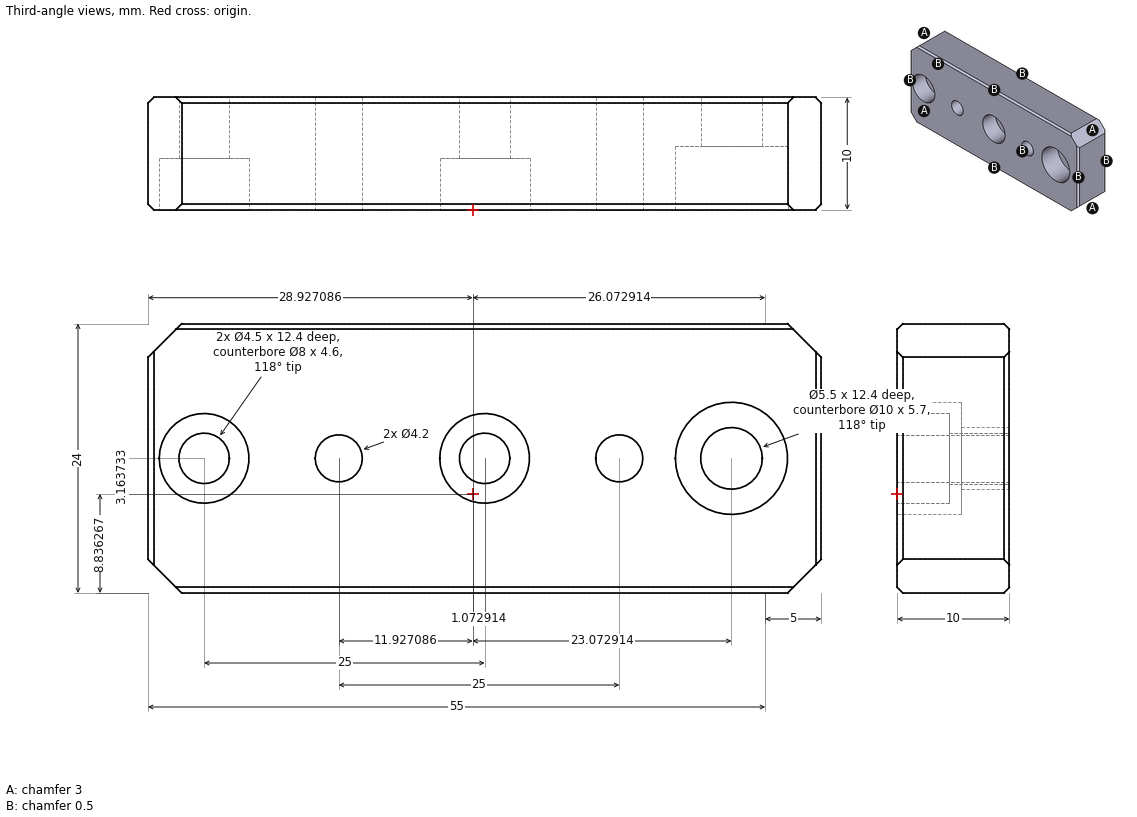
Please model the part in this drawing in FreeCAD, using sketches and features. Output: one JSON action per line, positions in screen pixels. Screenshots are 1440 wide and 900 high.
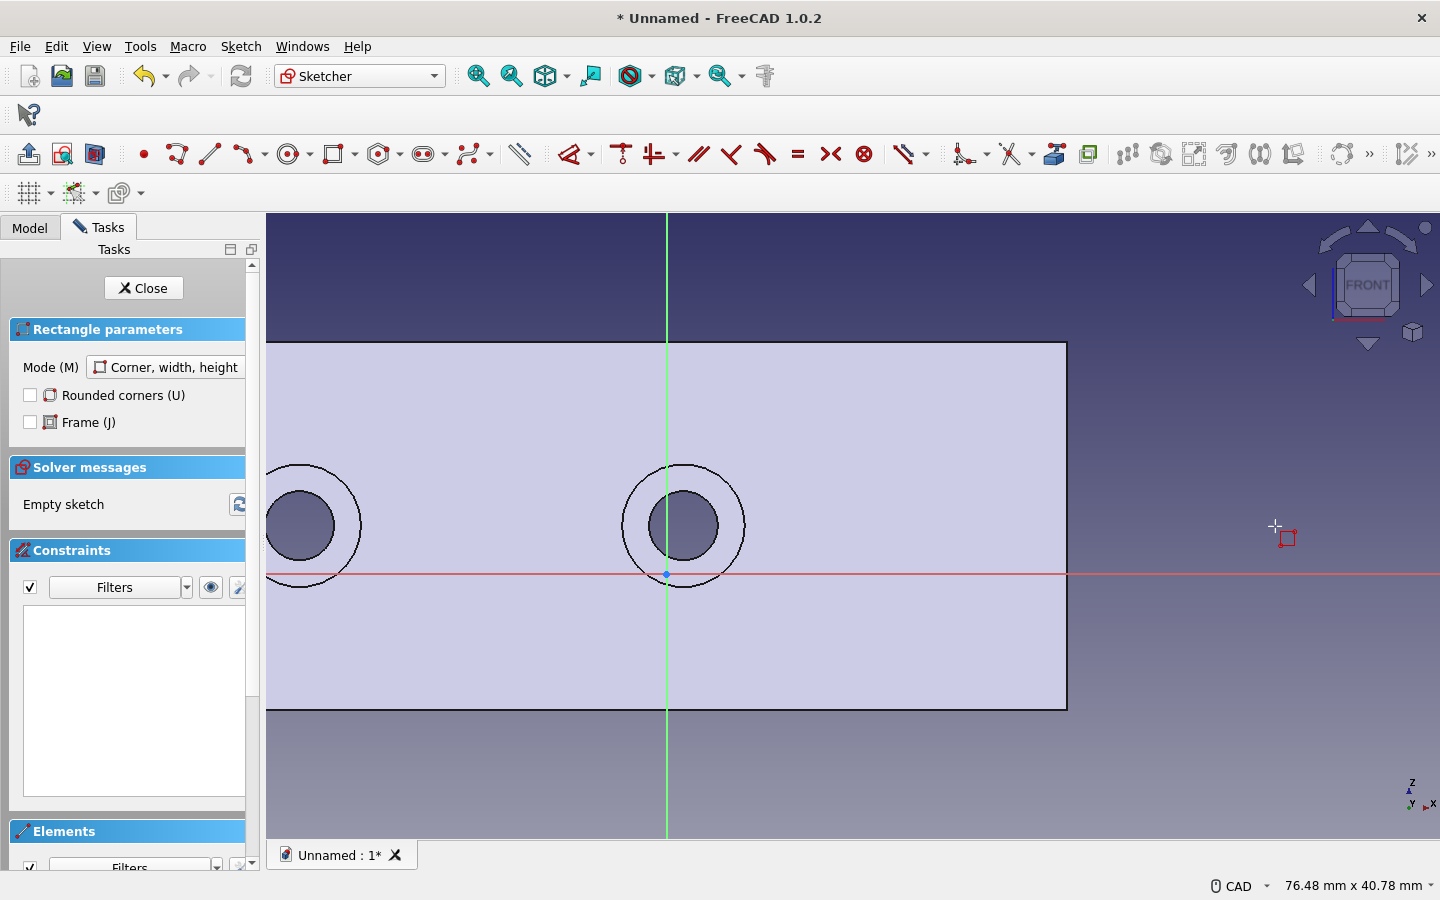
{"action": "left_click", "coordinate": [1067, 342]}
{"action": "left_click", "coordinate": [1144, 710]}
{"action": "key", "text": "Escape"}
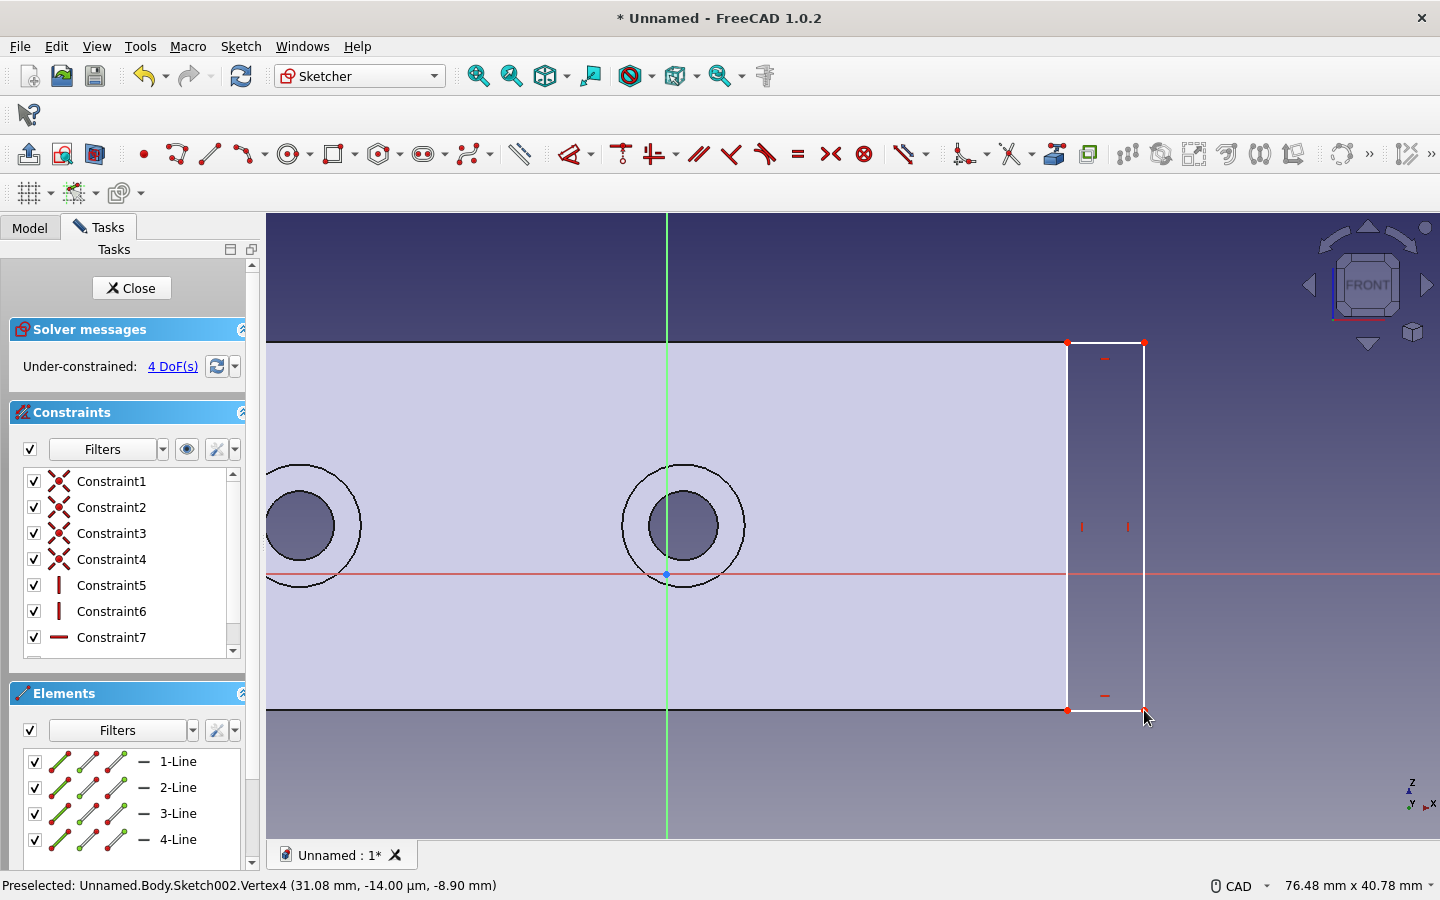
{"action": "key", "text": "d"}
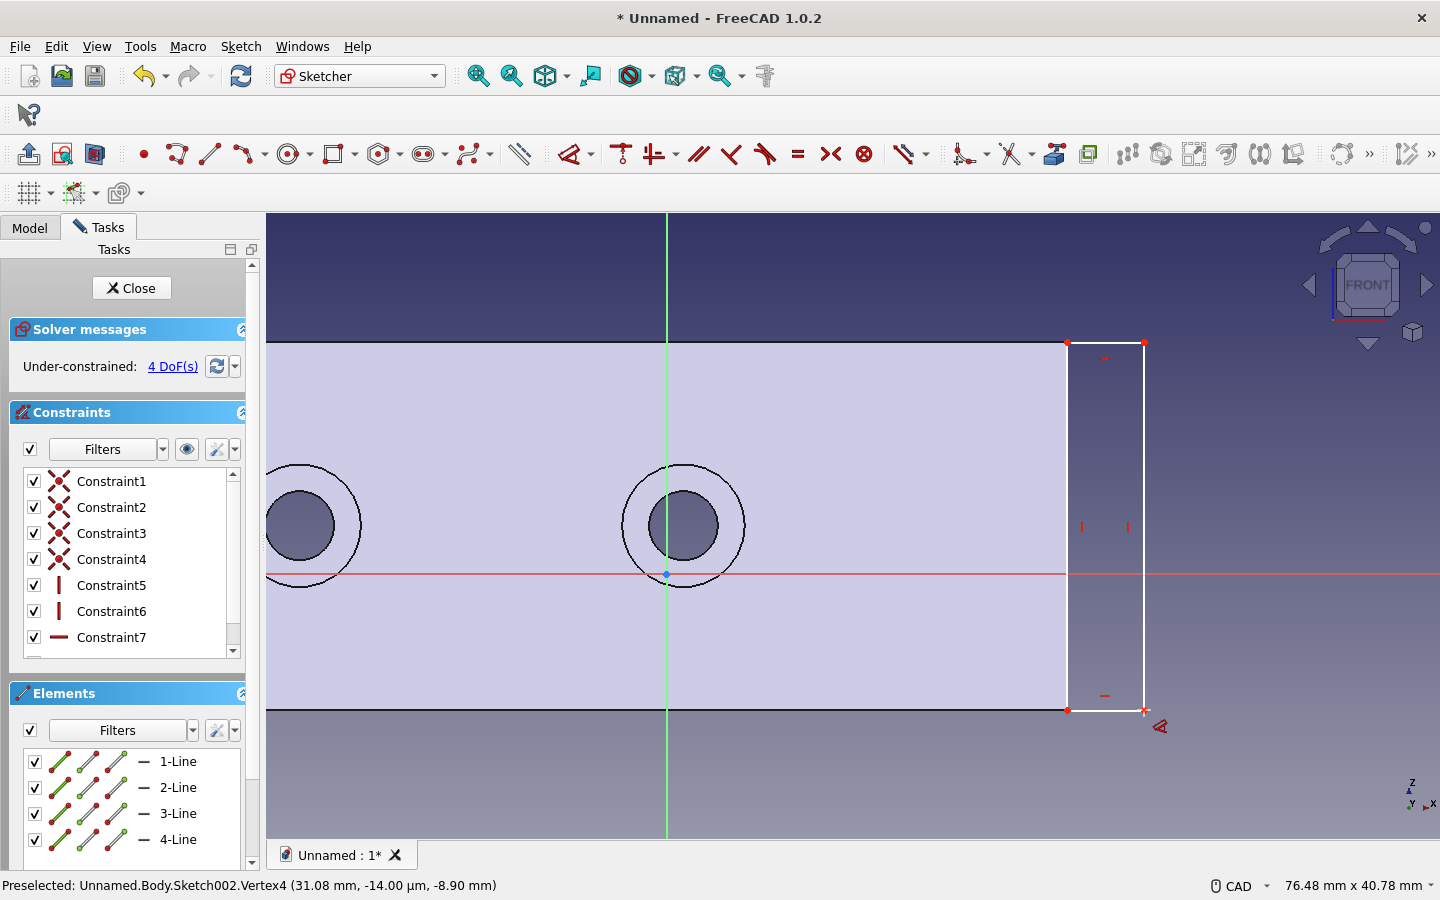
{"action": "left_click", "coordinate": [1090, 711]}
{"action": "left_click", "coordinate": [1105, 745]}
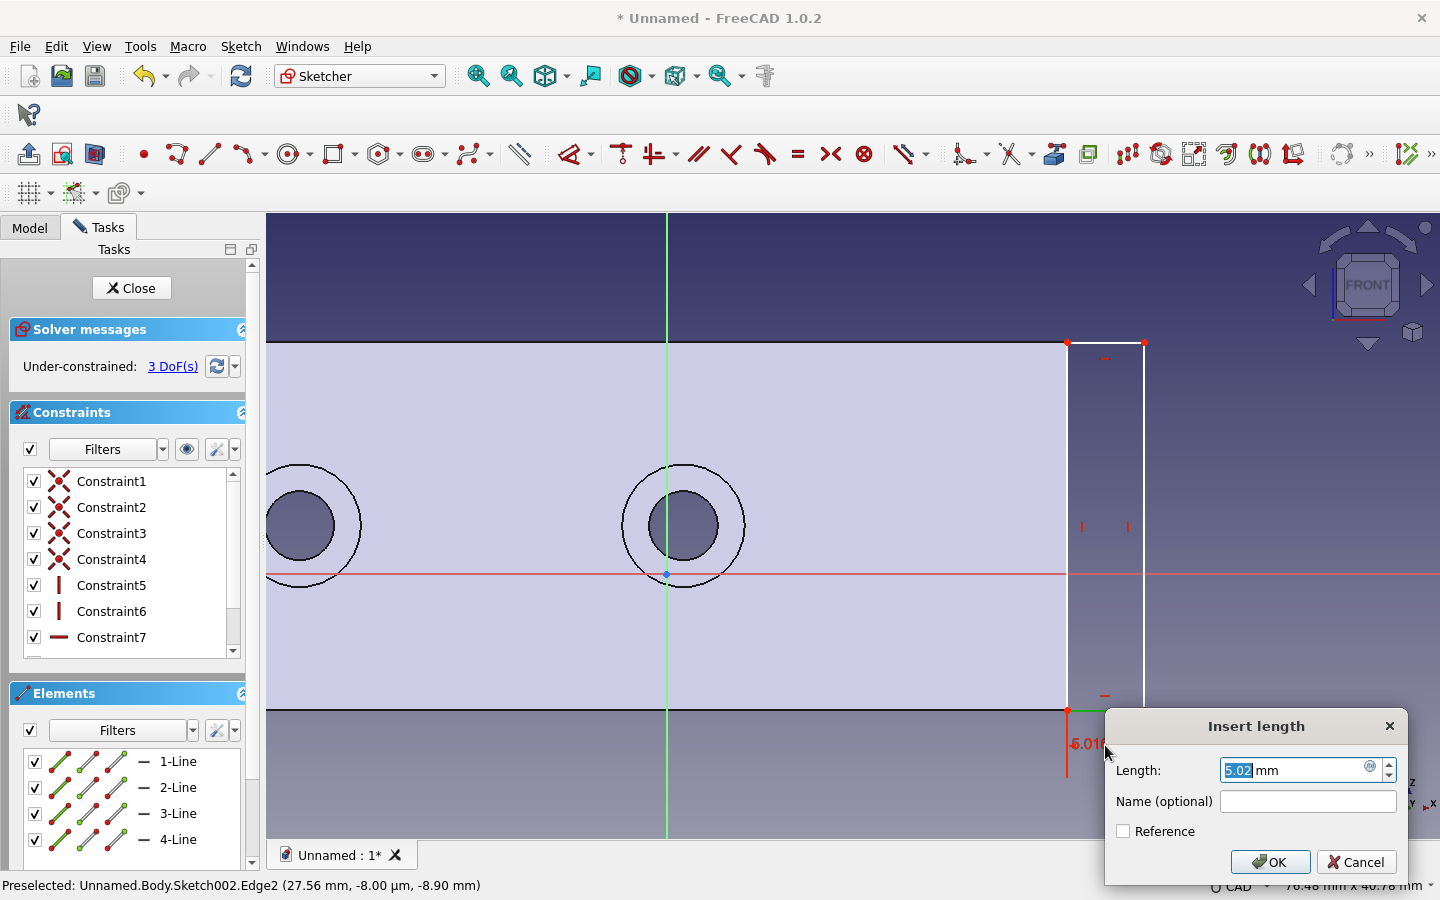
{"action": "type", "text": "5"}
{"action": "key", "text": "Return"}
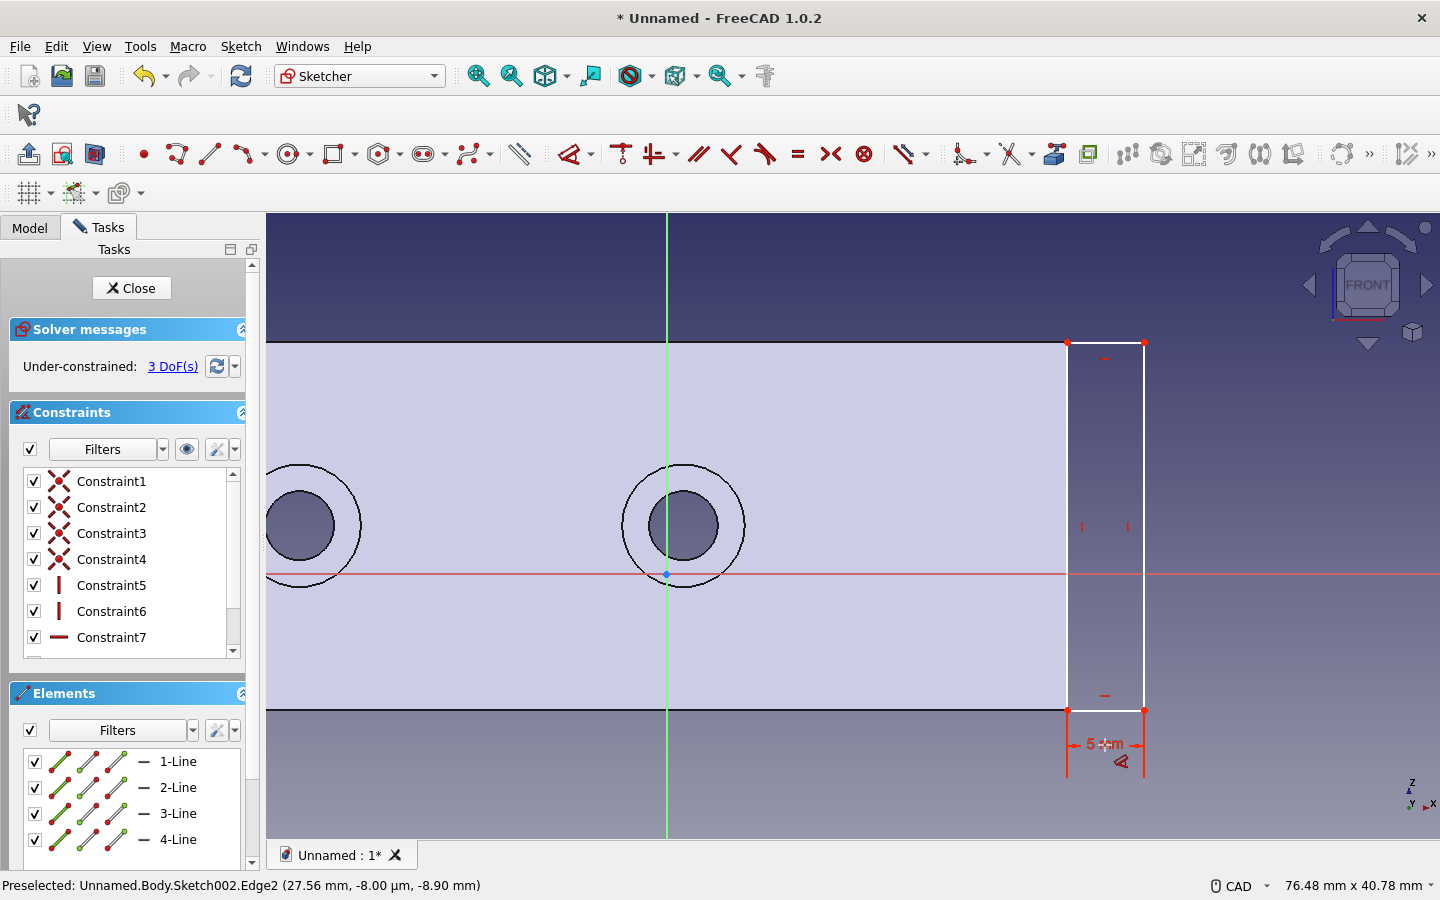
{"action": "left_click", "coordinate": [1067, 453]}
{"action": "left_click", "coordinate": [1101, 527]}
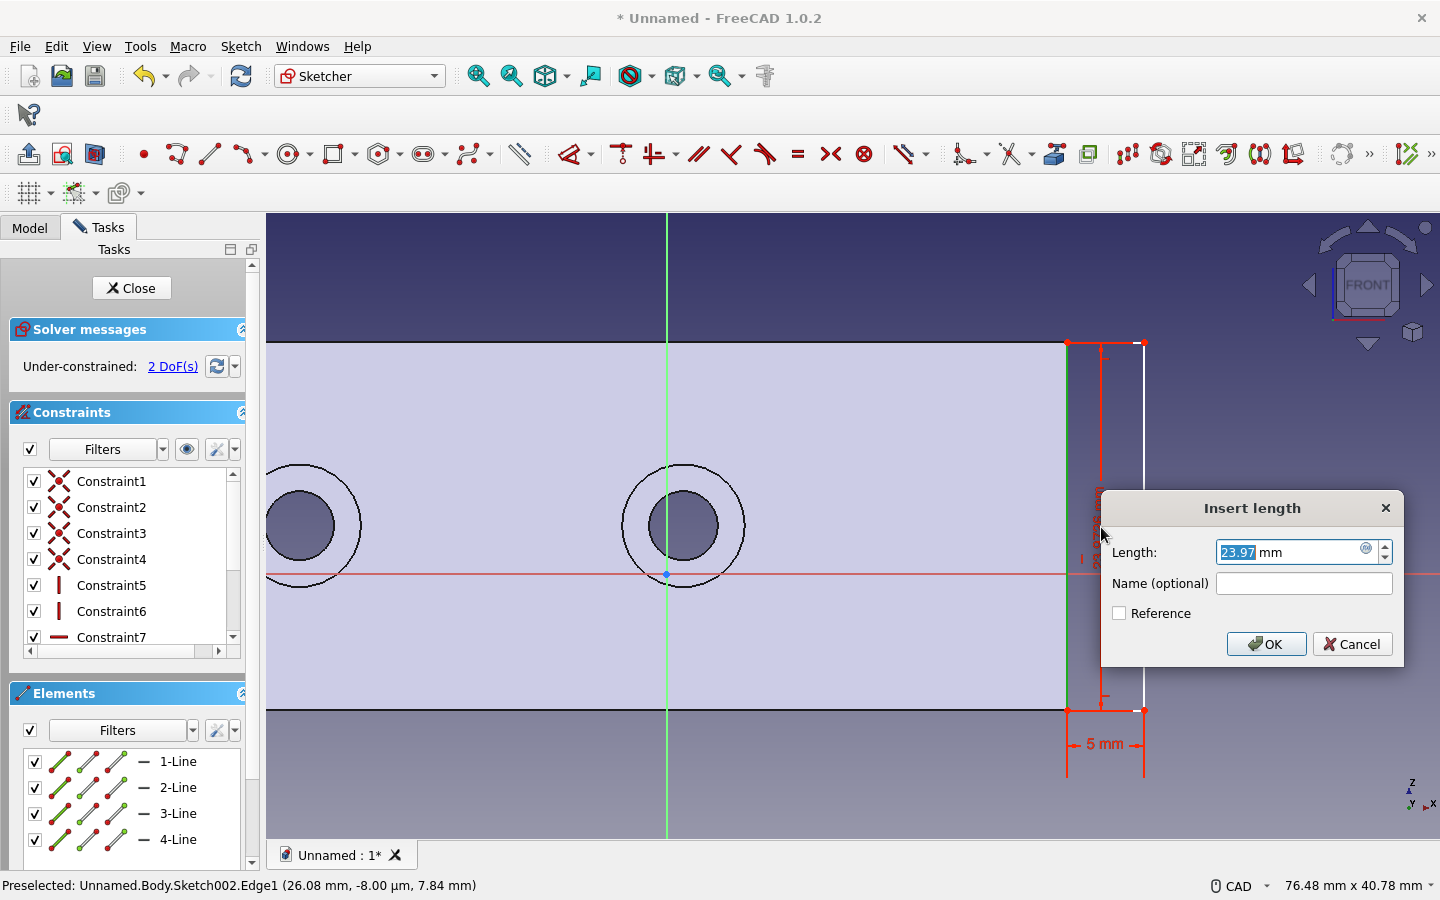
{"action": "type", "text": "24"}
{"action": "key", "text": "Return"}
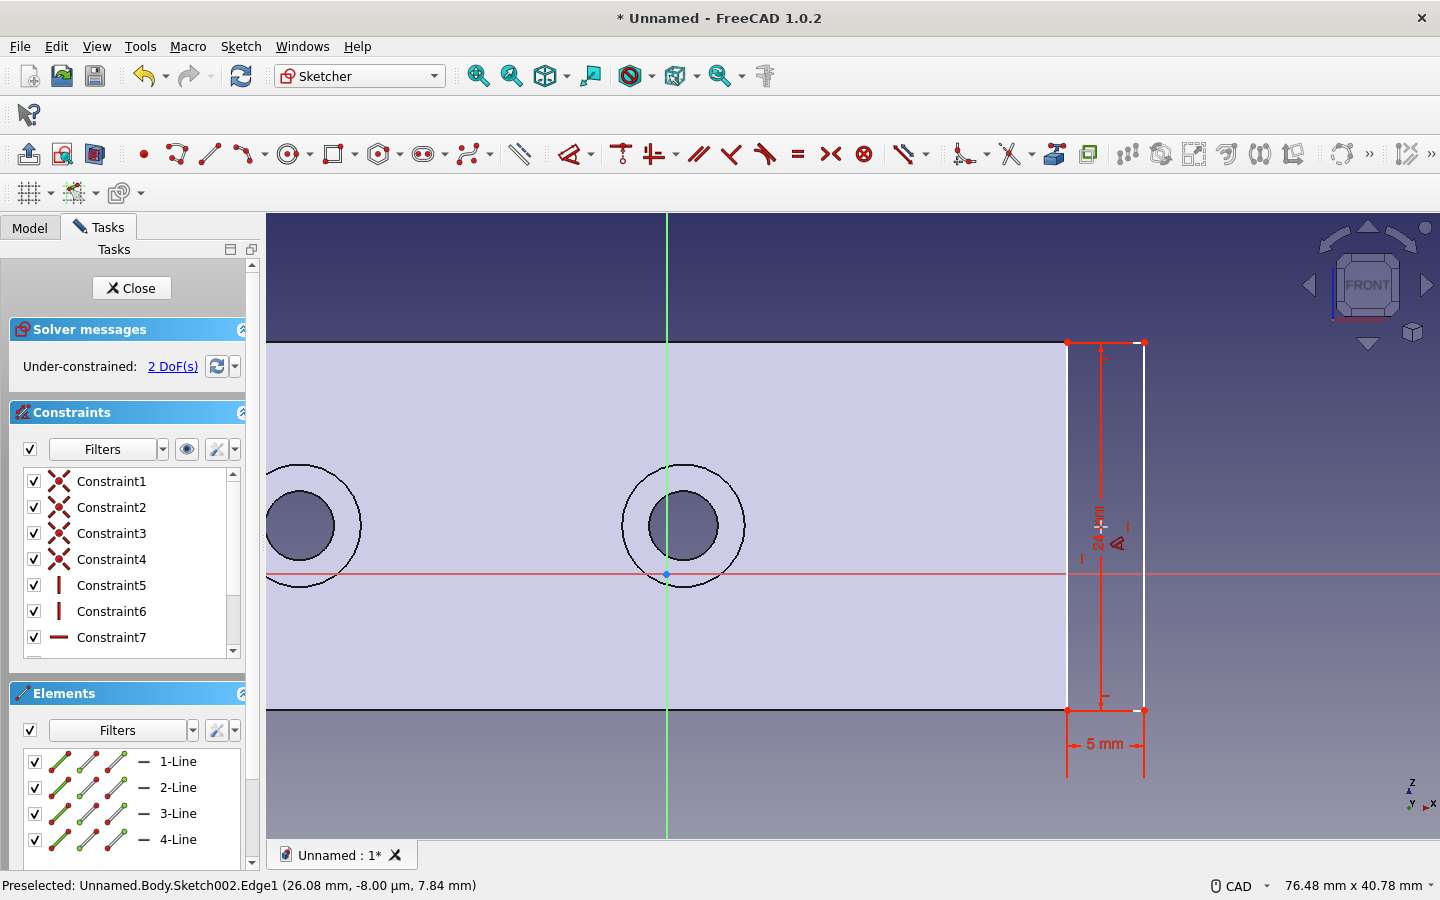
{"action": "left_click", "coordinate": [1067, 711]}
{"action": "left_click", "coordinate": [633, 643]}